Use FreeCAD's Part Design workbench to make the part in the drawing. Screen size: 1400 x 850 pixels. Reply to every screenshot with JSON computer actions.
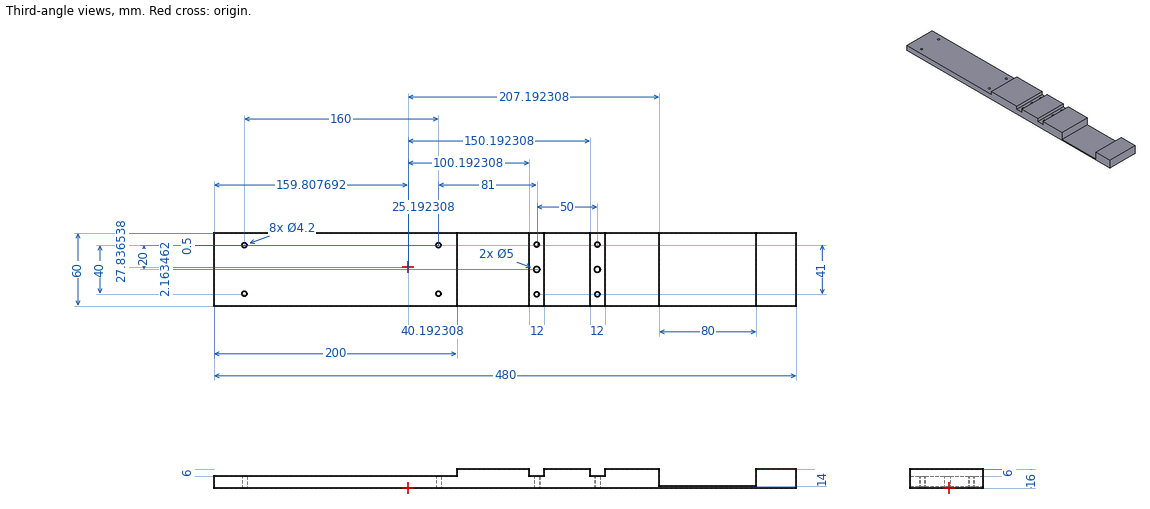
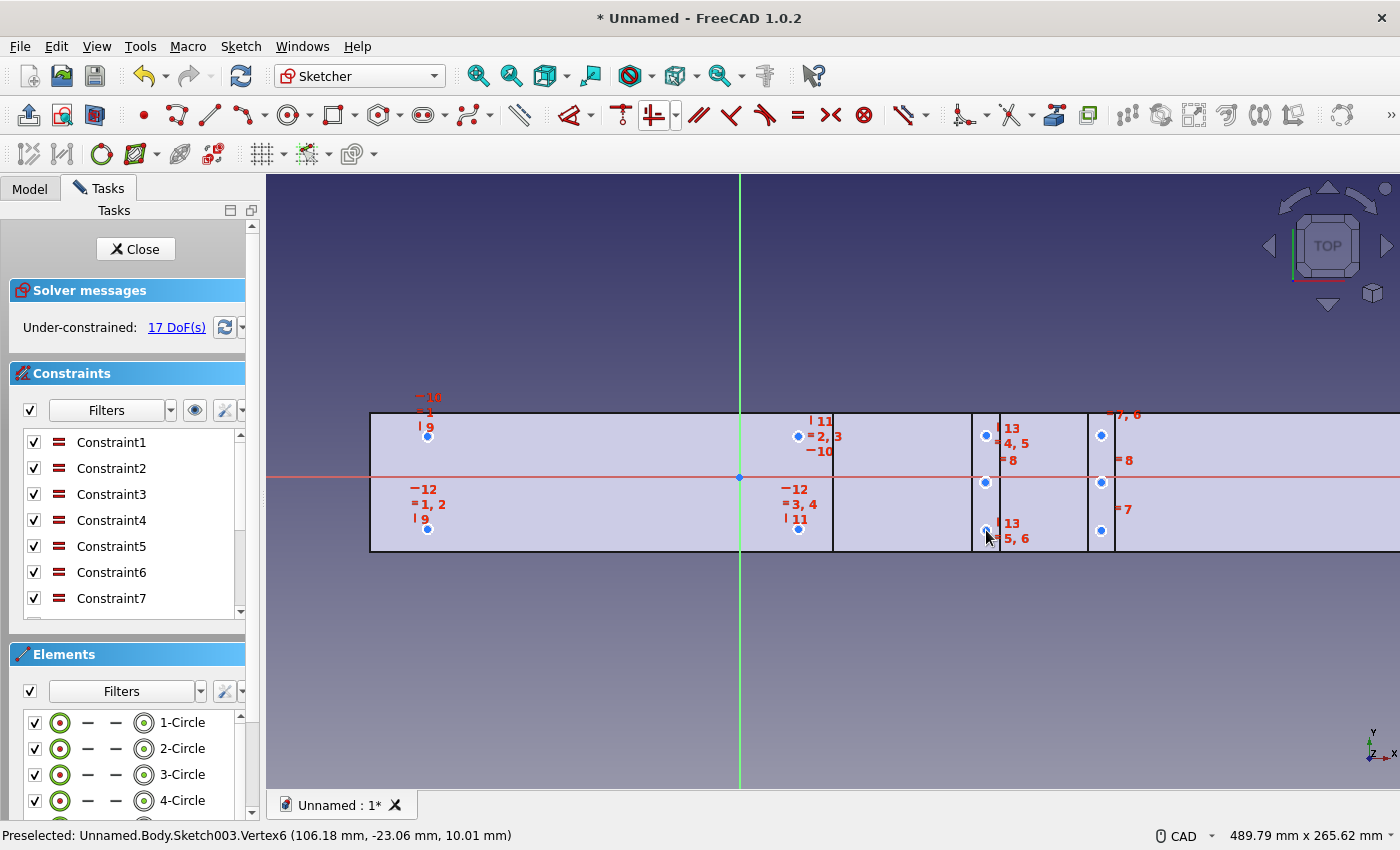
{"action": "left_click", "coordinate": [986, 436]}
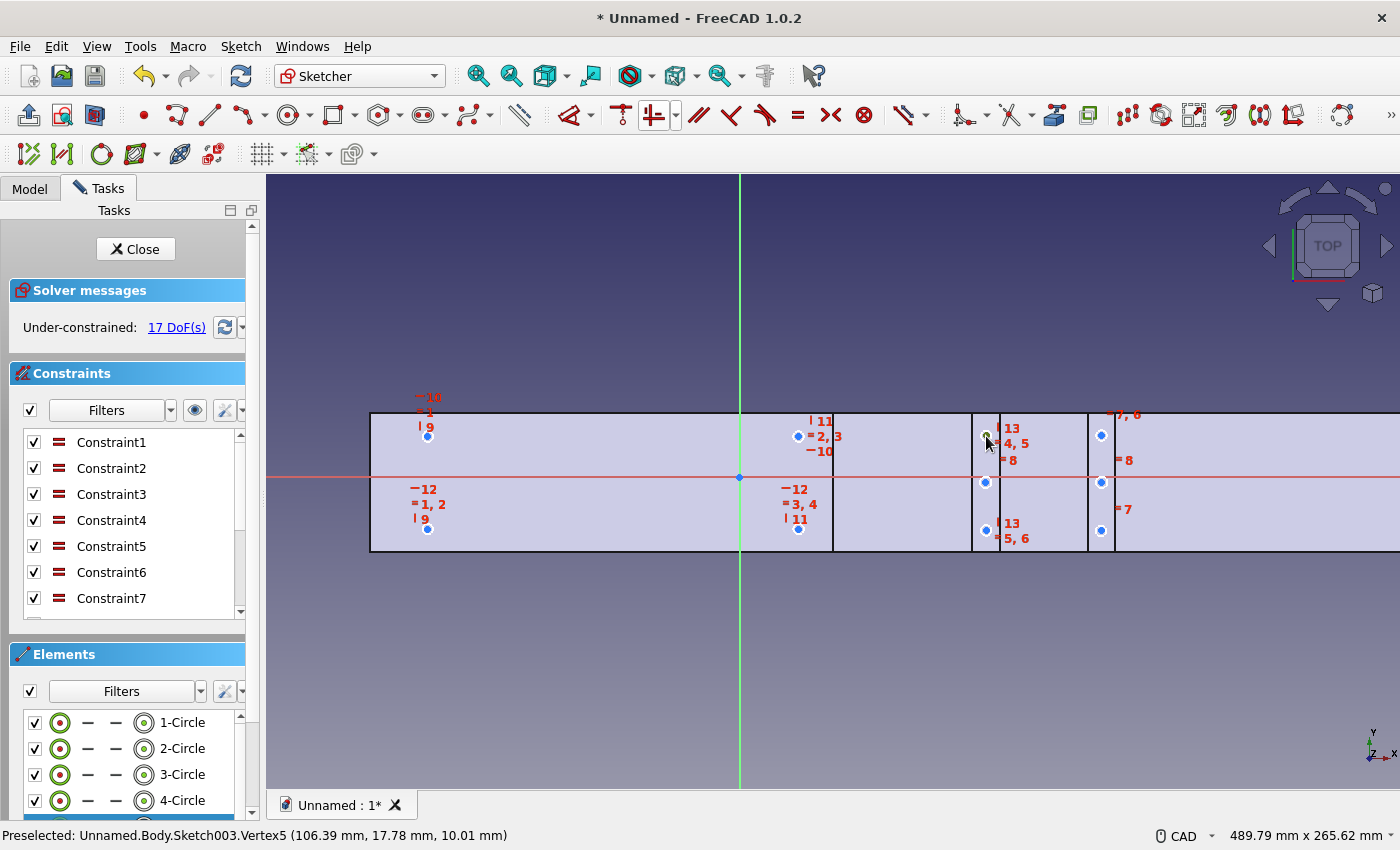
{"action": "left_click", "coordinate": [1102, 435]}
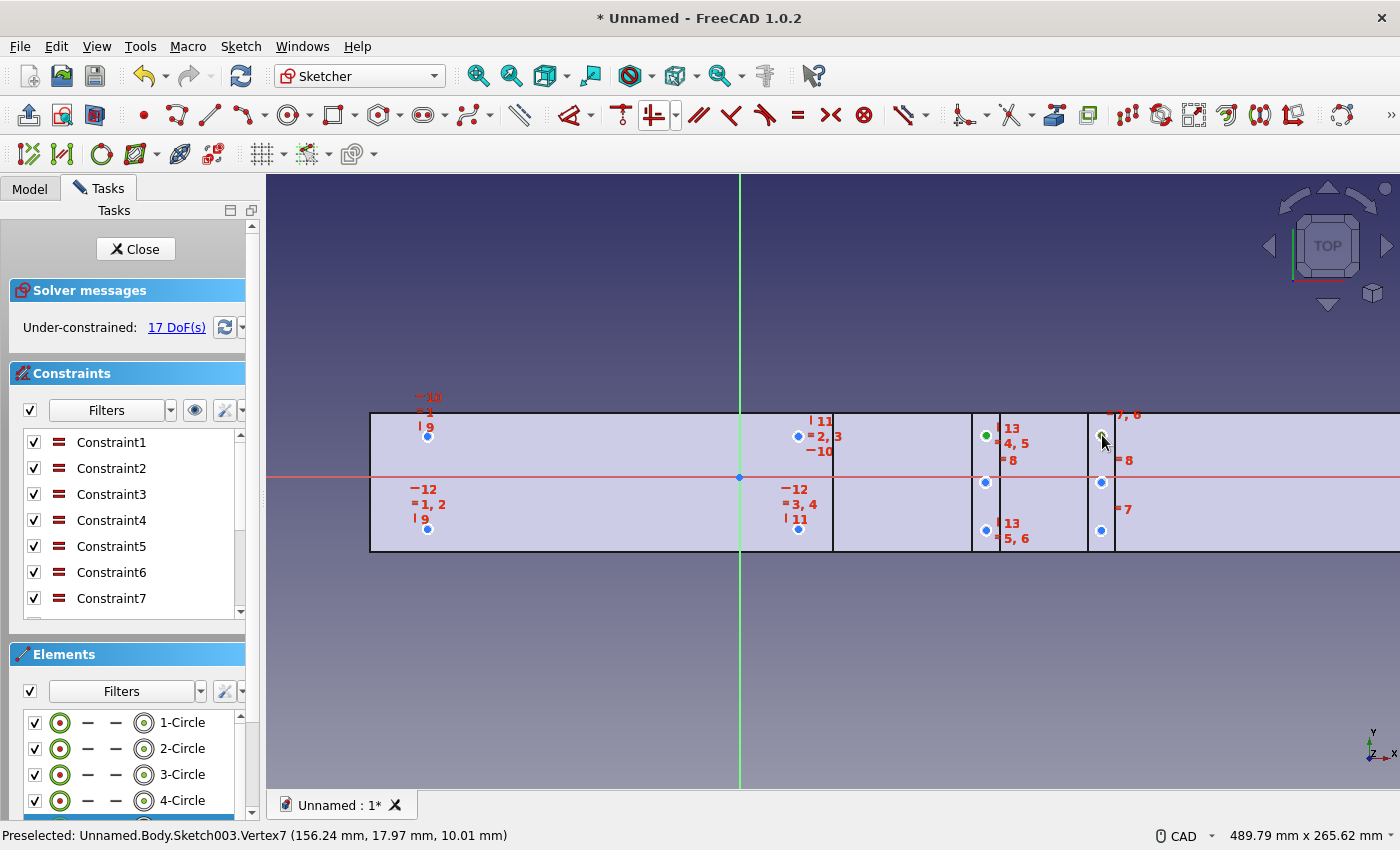
{"action": "key", "text": "h"}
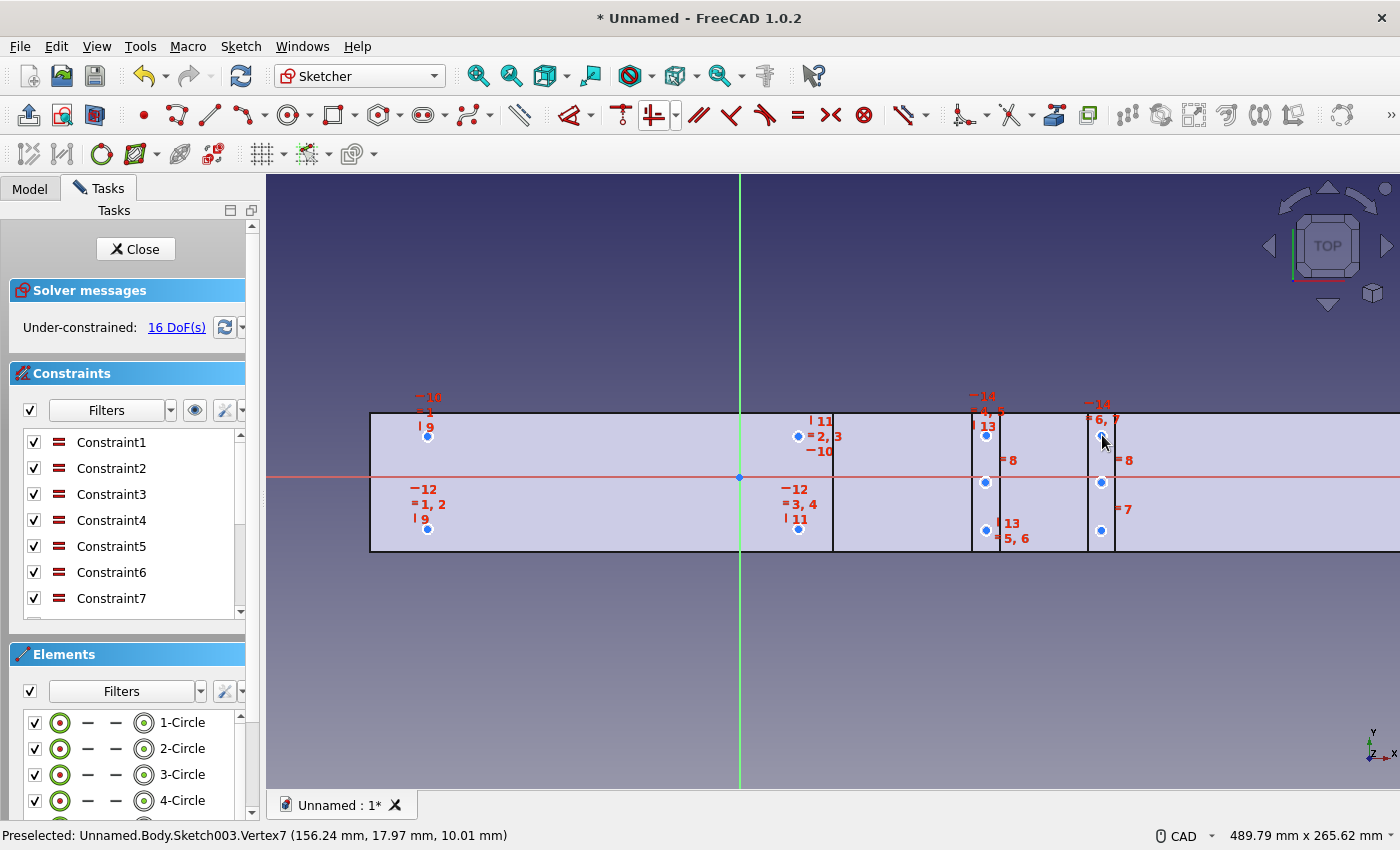
{"action": "left_click", "coordinate": [1102, 436]}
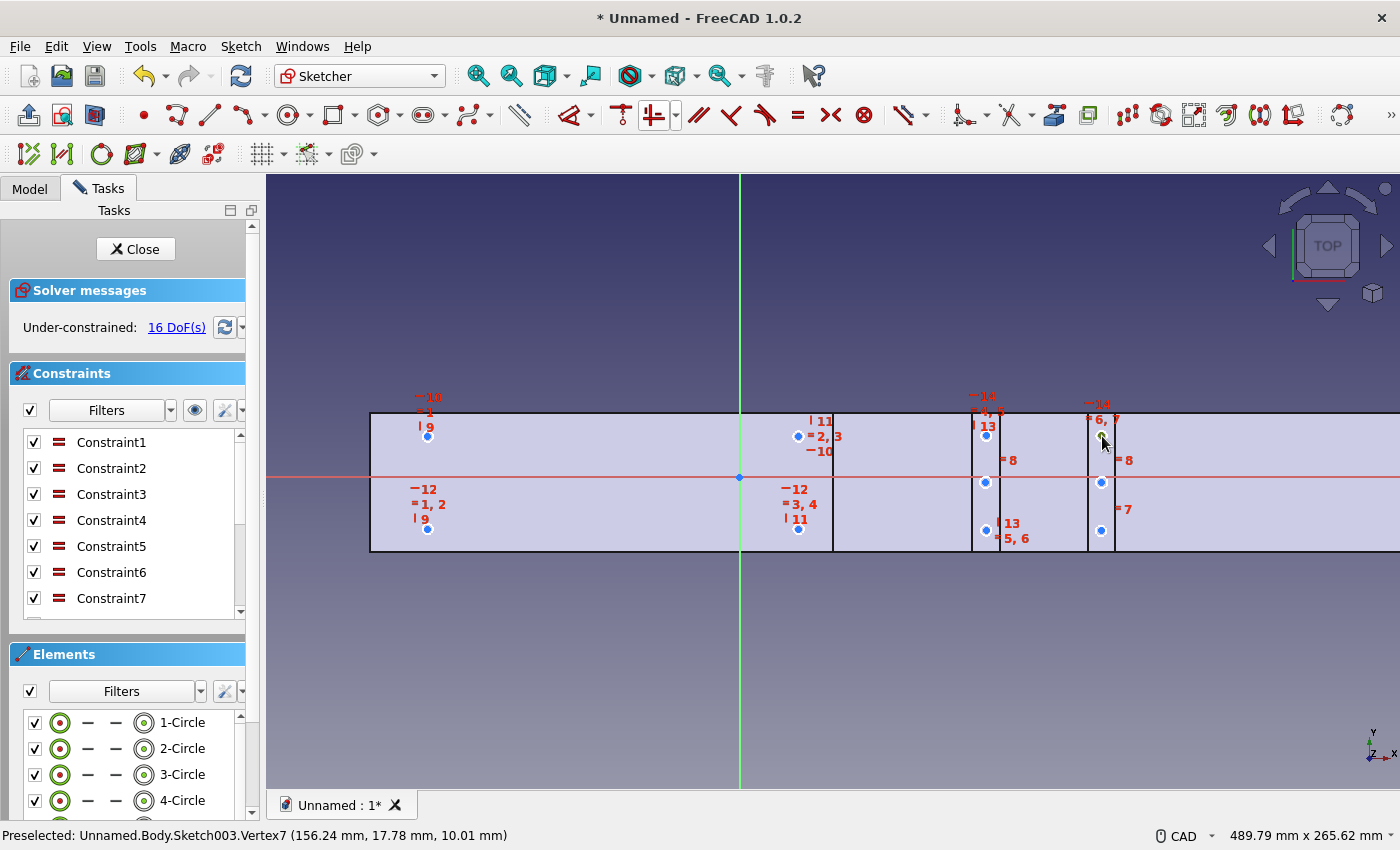
{"action": "left_click", "coordinate": [1101, 531]}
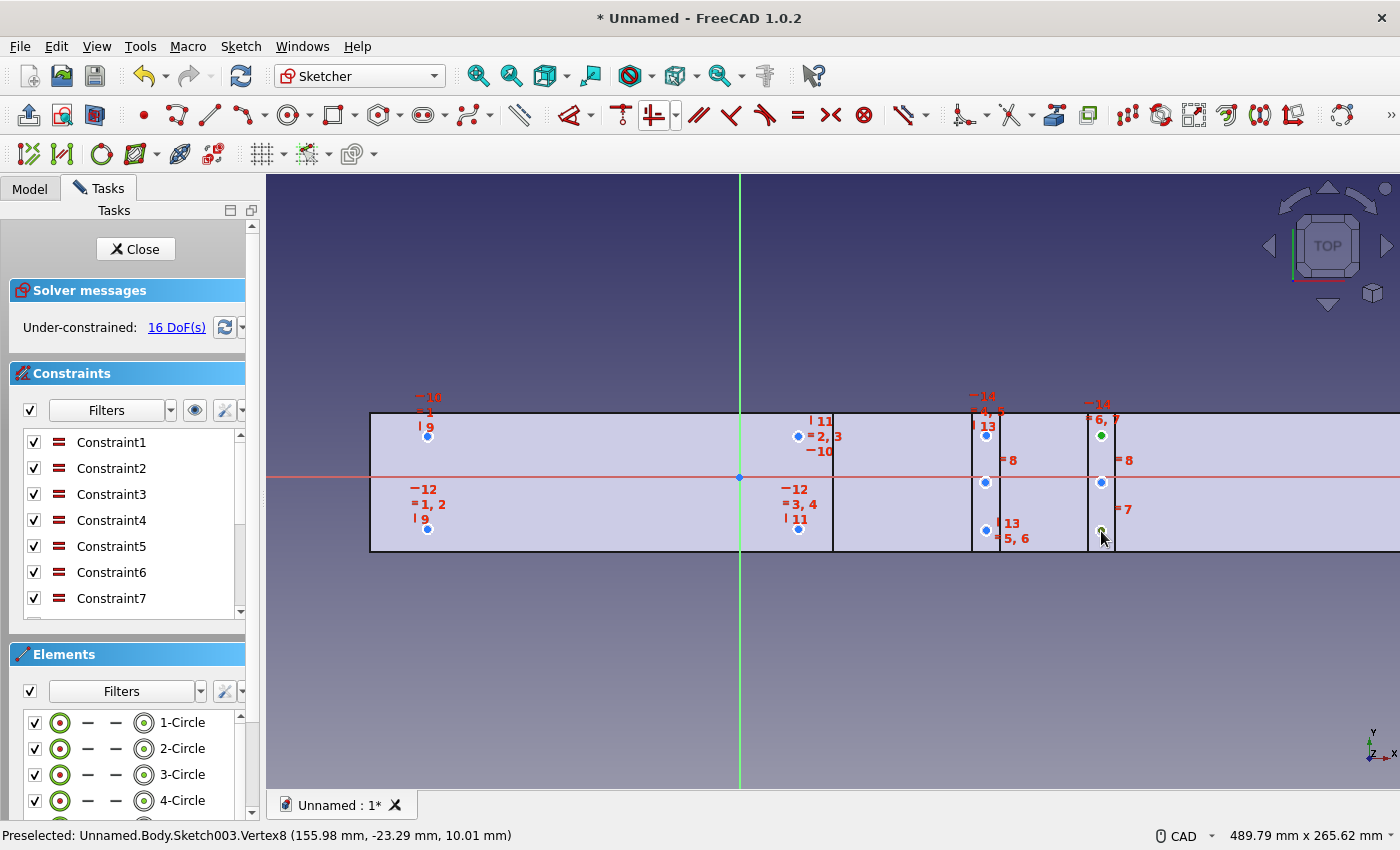
{"action": "left_click", "coordinate": [676, 116]}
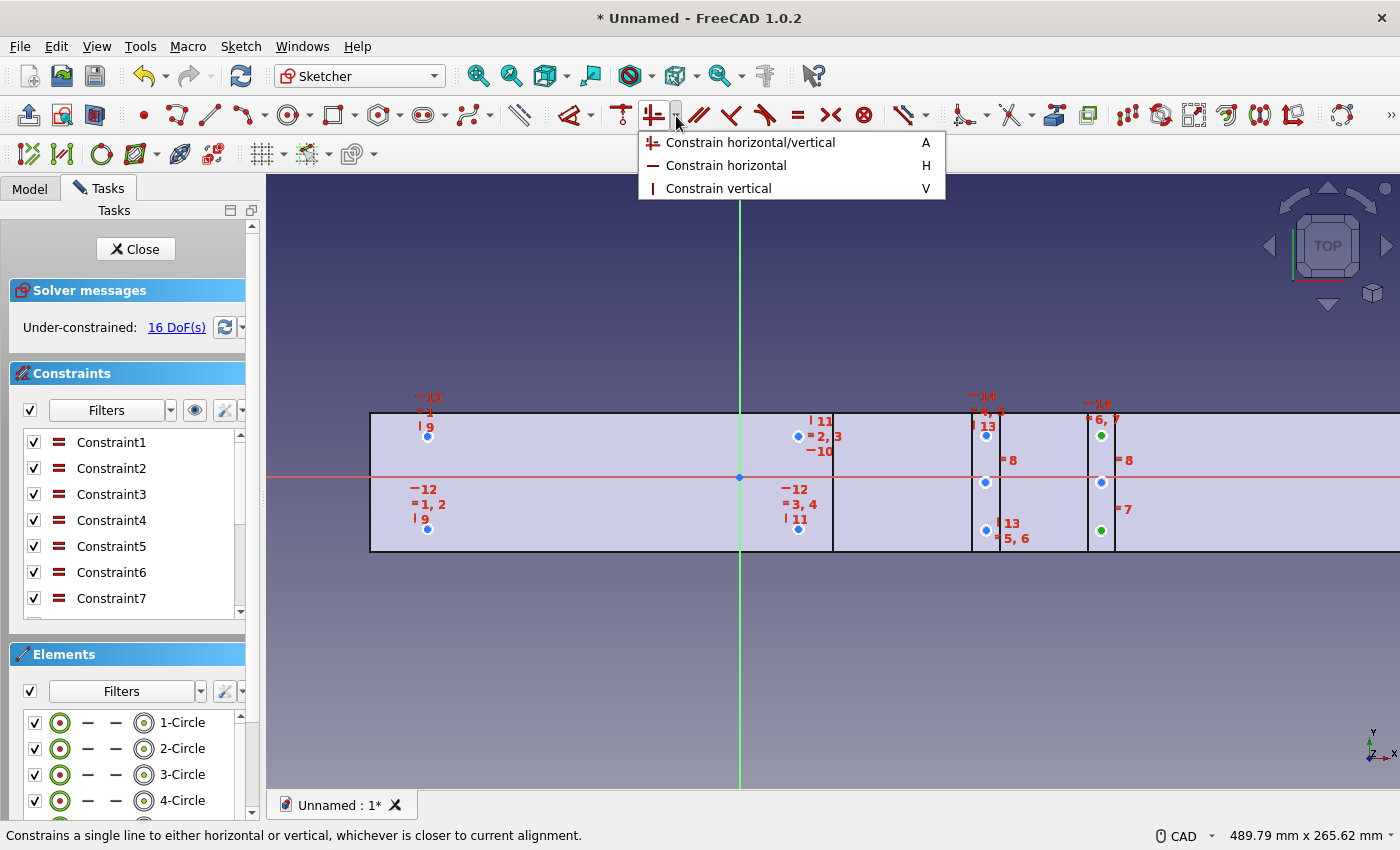
{"action": "left_click", "coordinate": [792, 188]}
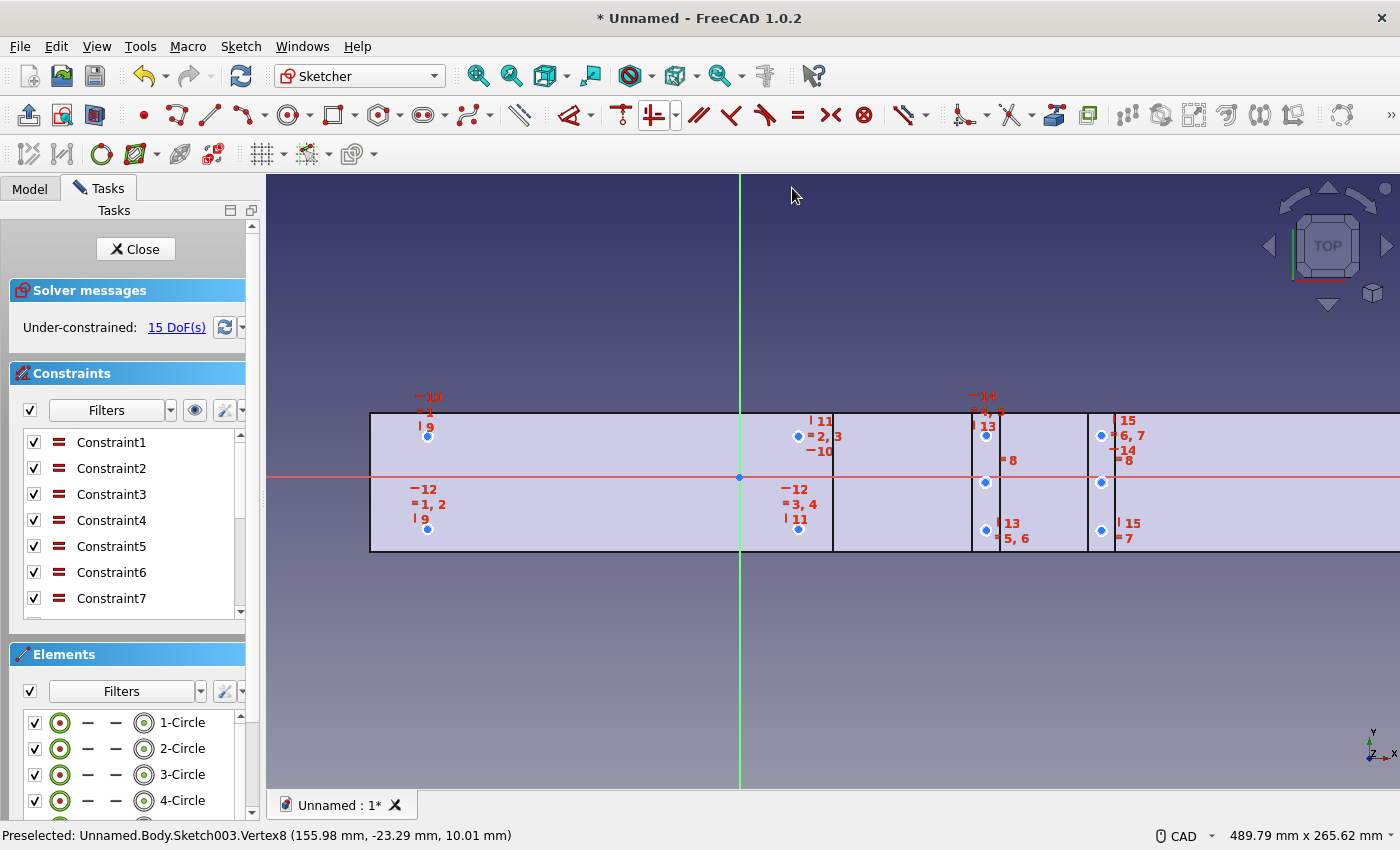
{"action": "left_click", "coordinate": [986, 530]}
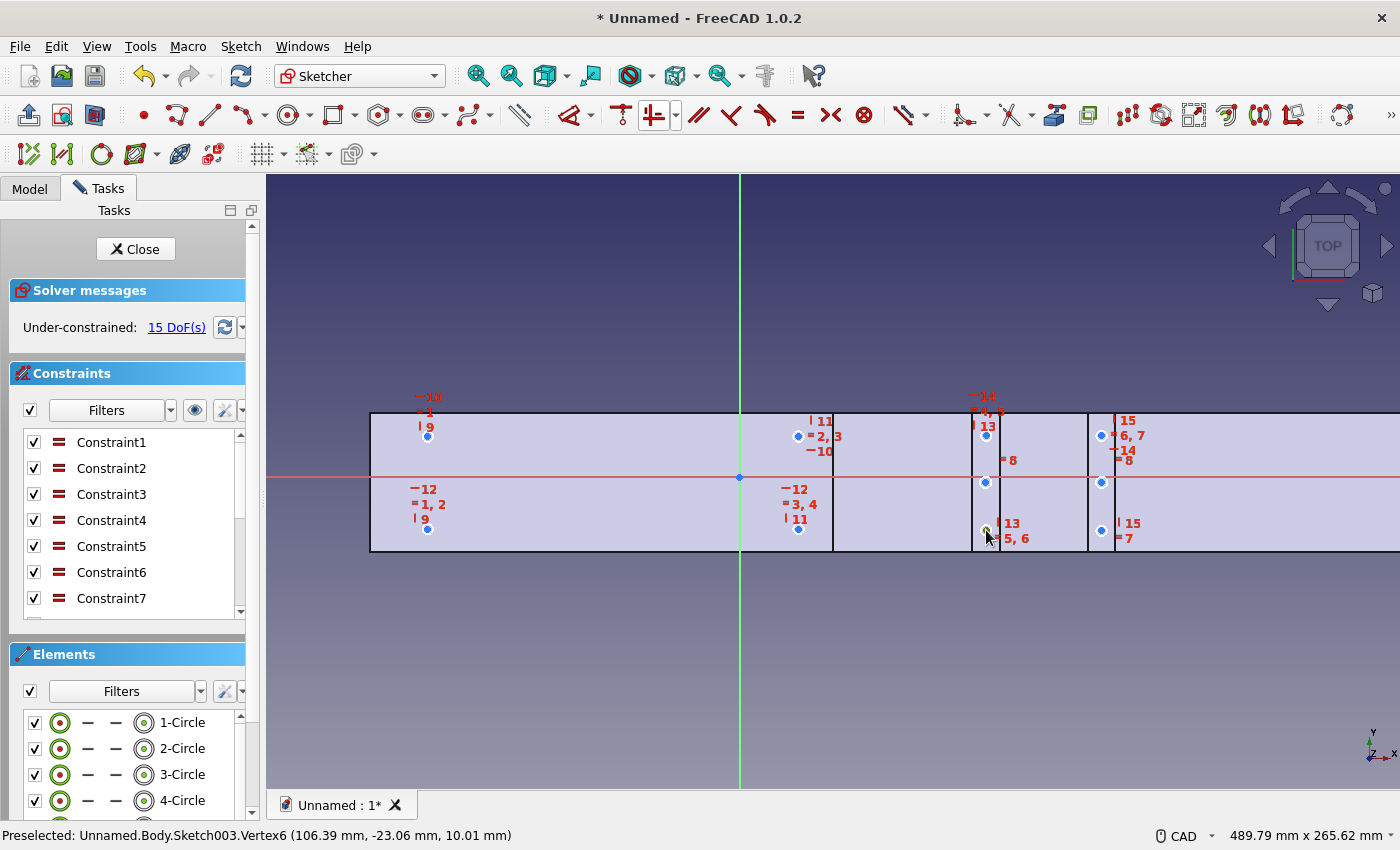
{"action": "left_click", "coordinate": [1102, 531]}